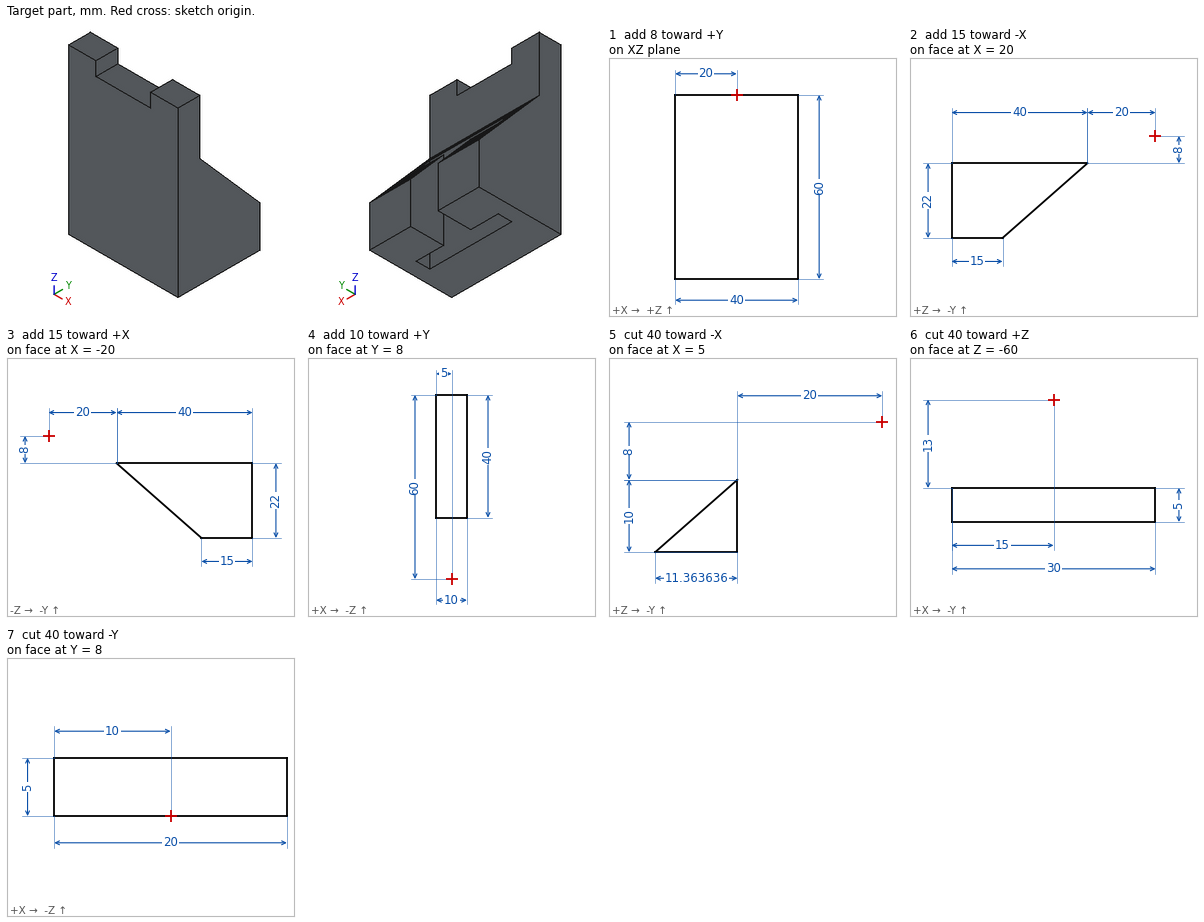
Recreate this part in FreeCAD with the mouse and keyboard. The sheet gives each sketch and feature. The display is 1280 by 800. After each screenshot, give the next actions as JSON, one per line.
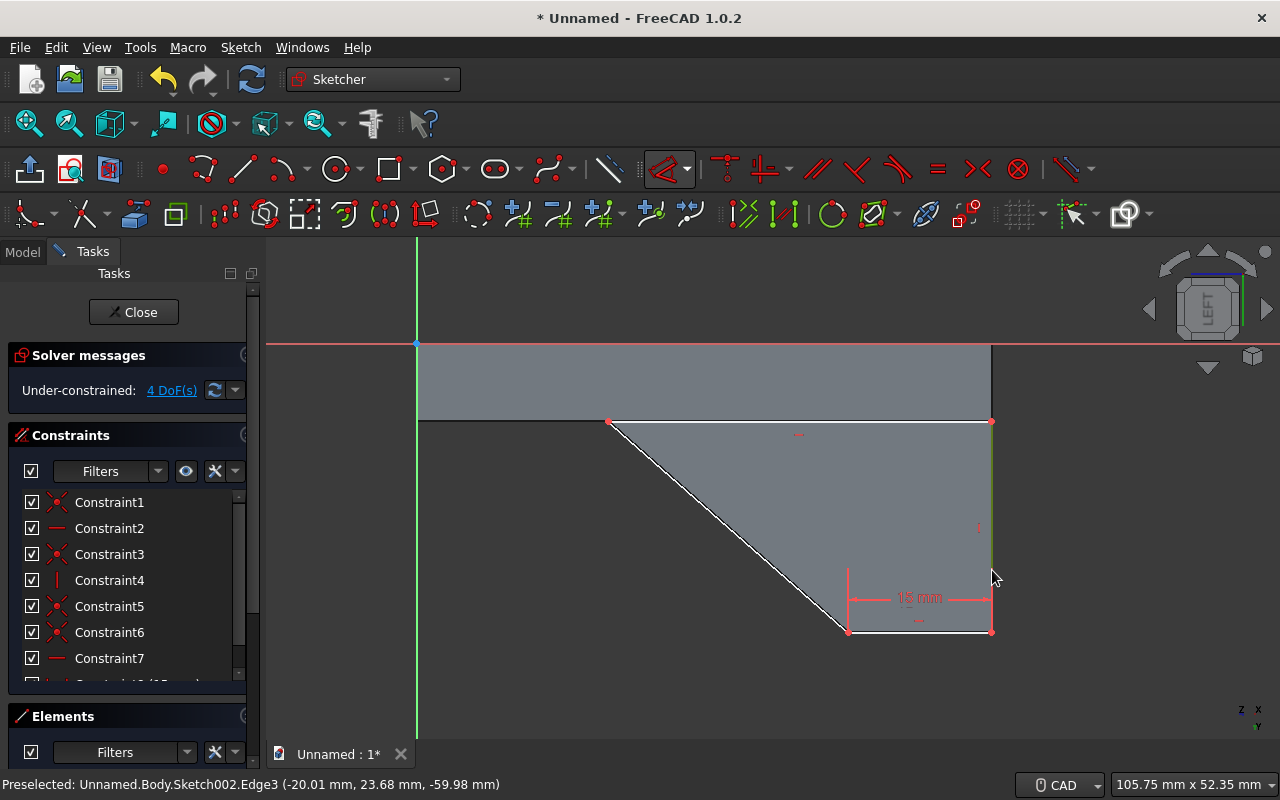
{"action": "left_click", "coordinate": [690, 170]}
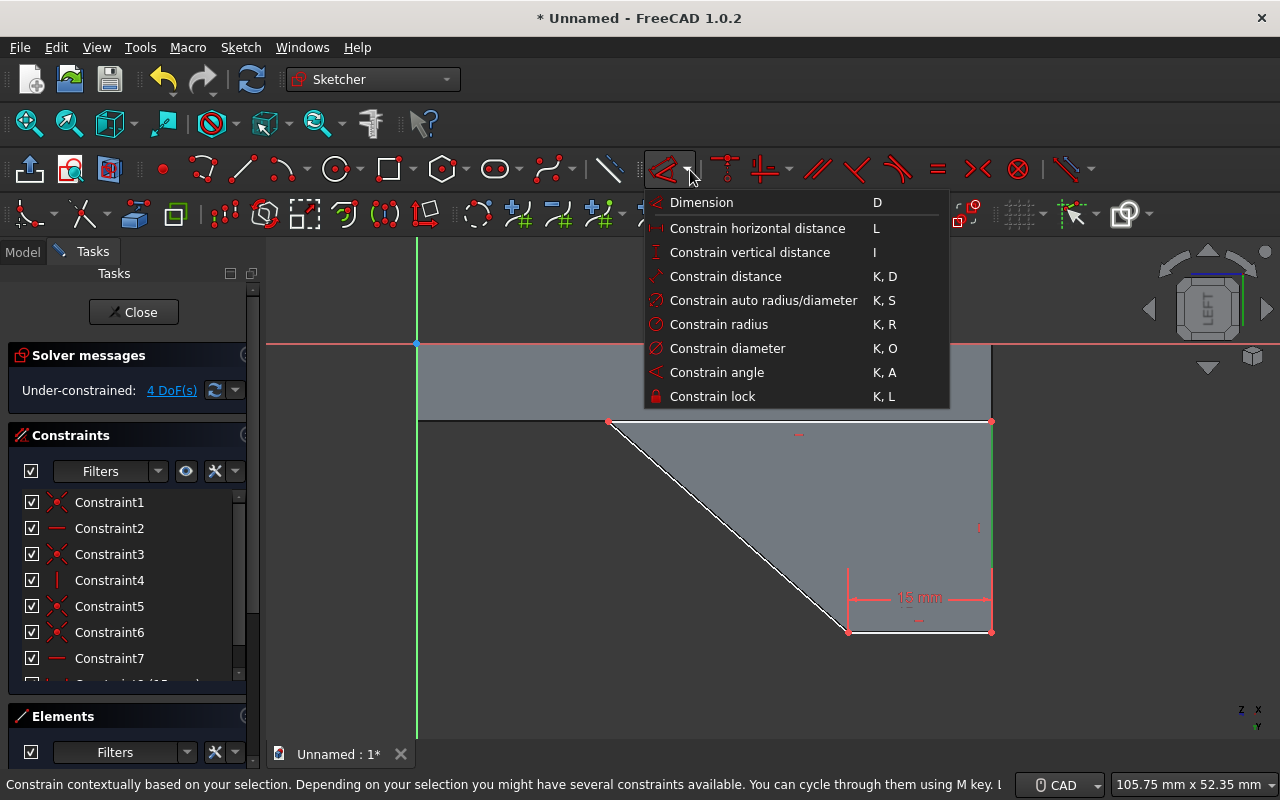
{"action": "left_click", "coordinate": [797, 252]}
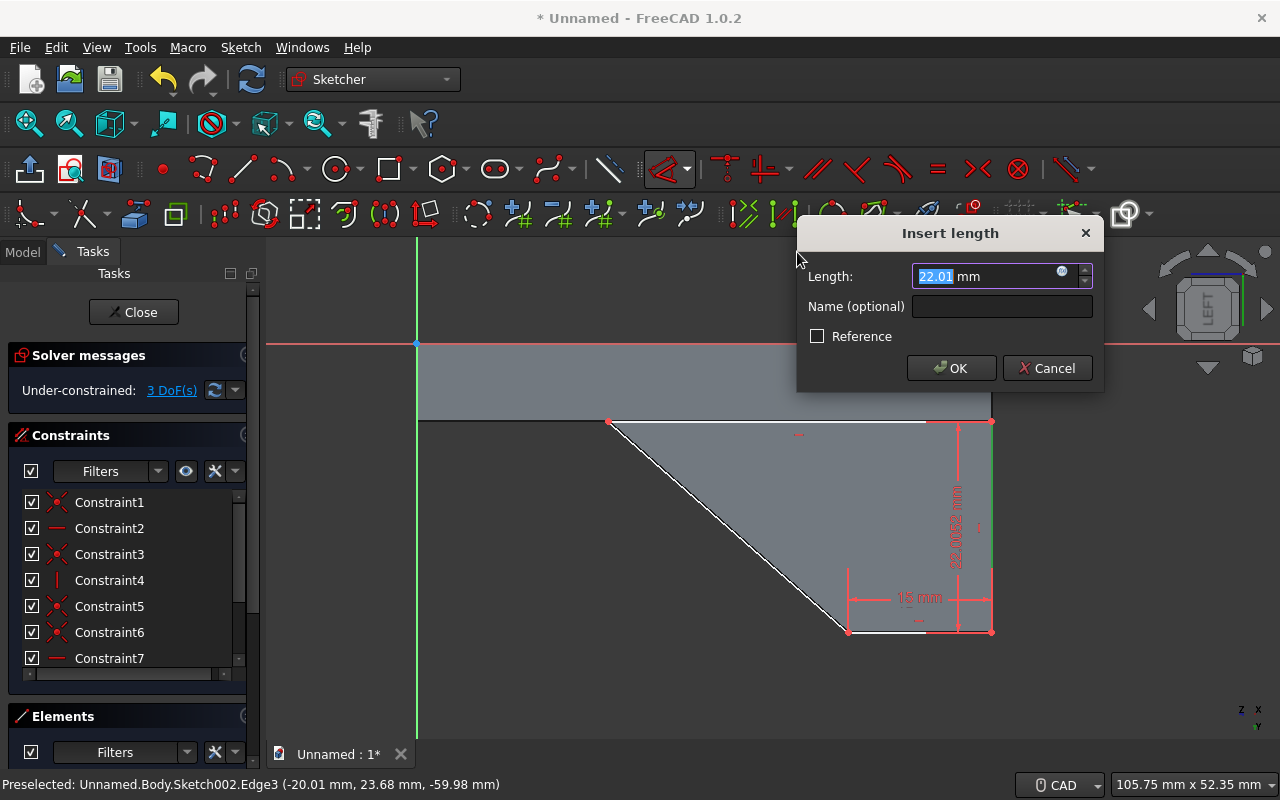
{"action": "type", "text": "22"}
{"action": "key", "text": "Return"}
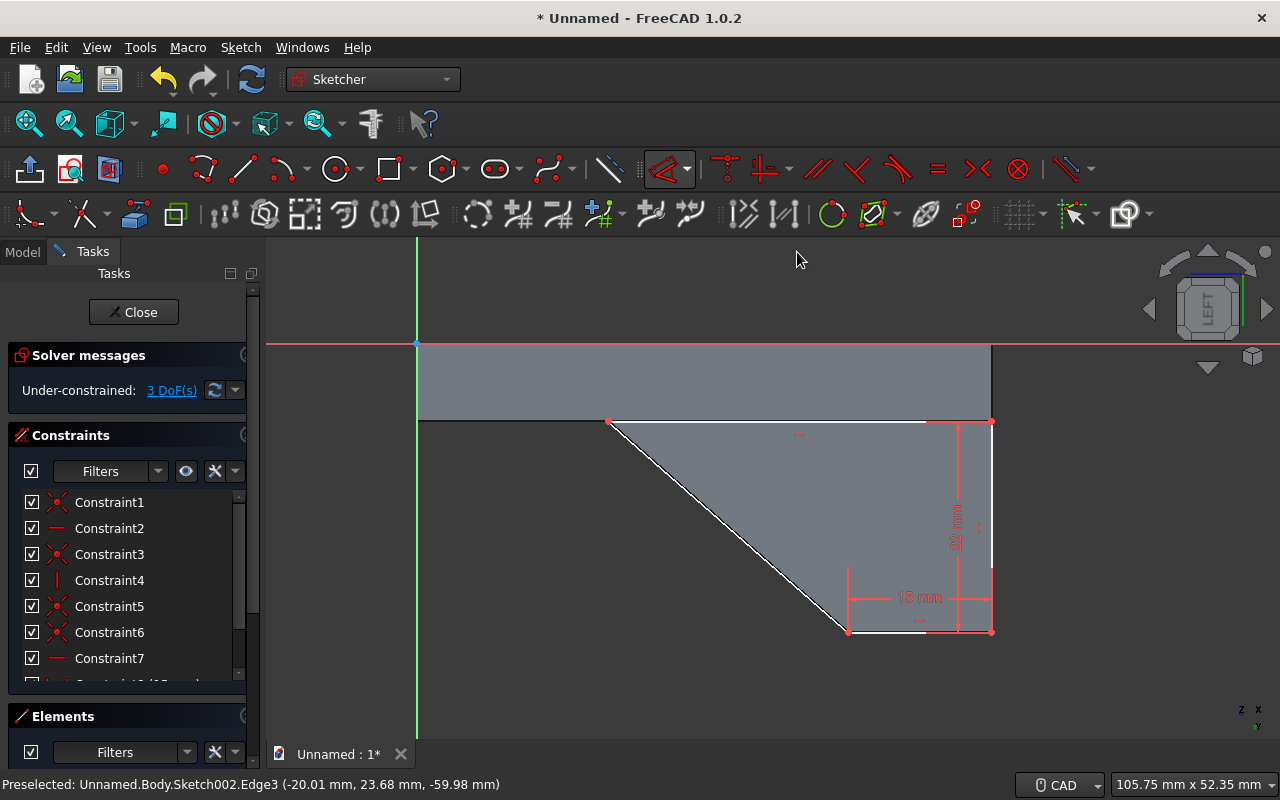
{"action": "left_click", "coordinate": [877, 422]}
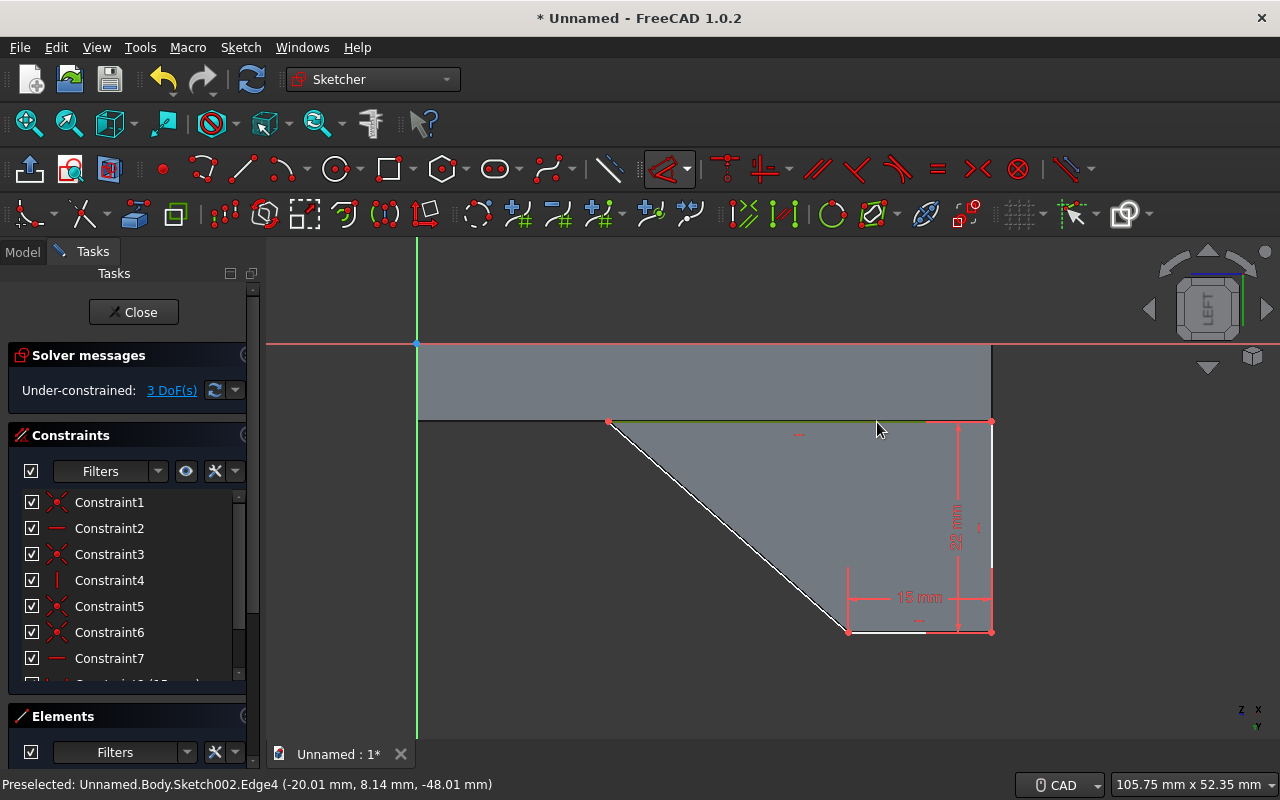
{"action": "left_click", "coordinate": [690, 170]}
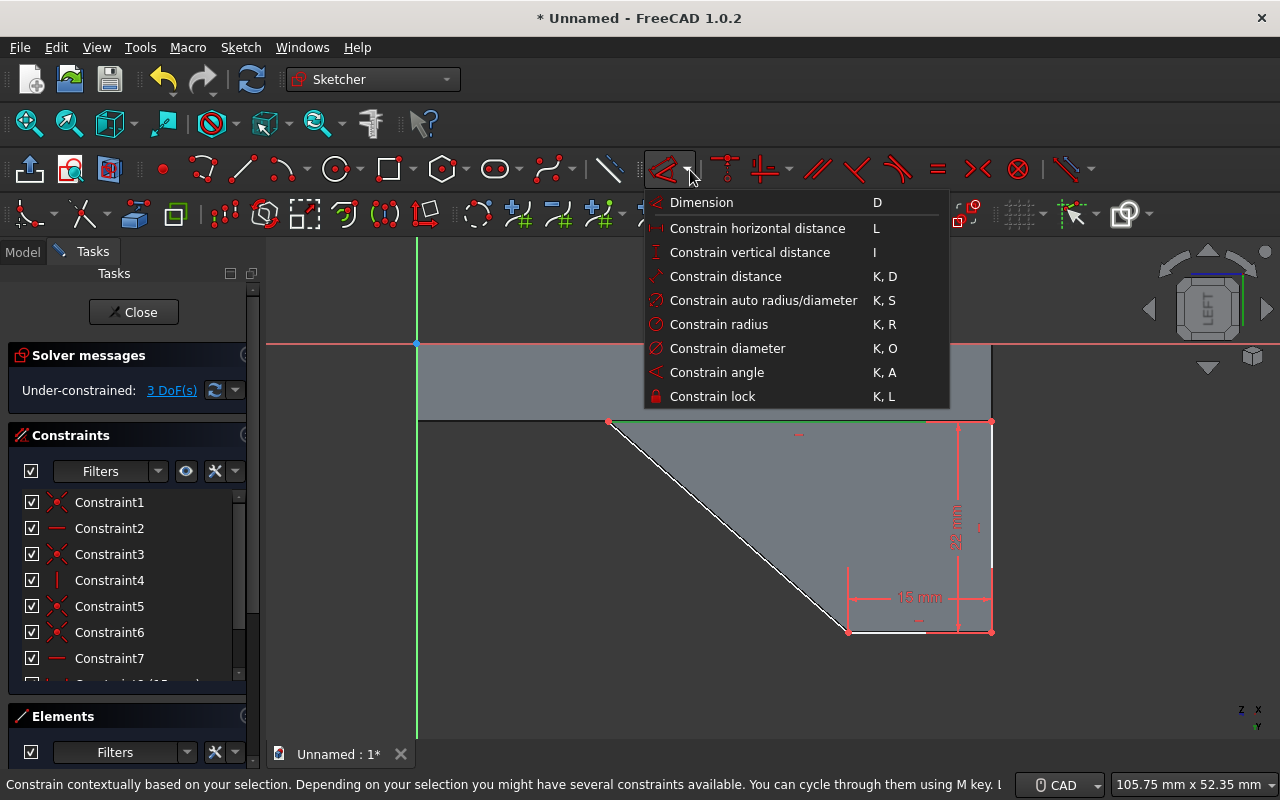
{"action": "left_click", "coordinate": [797, 228]}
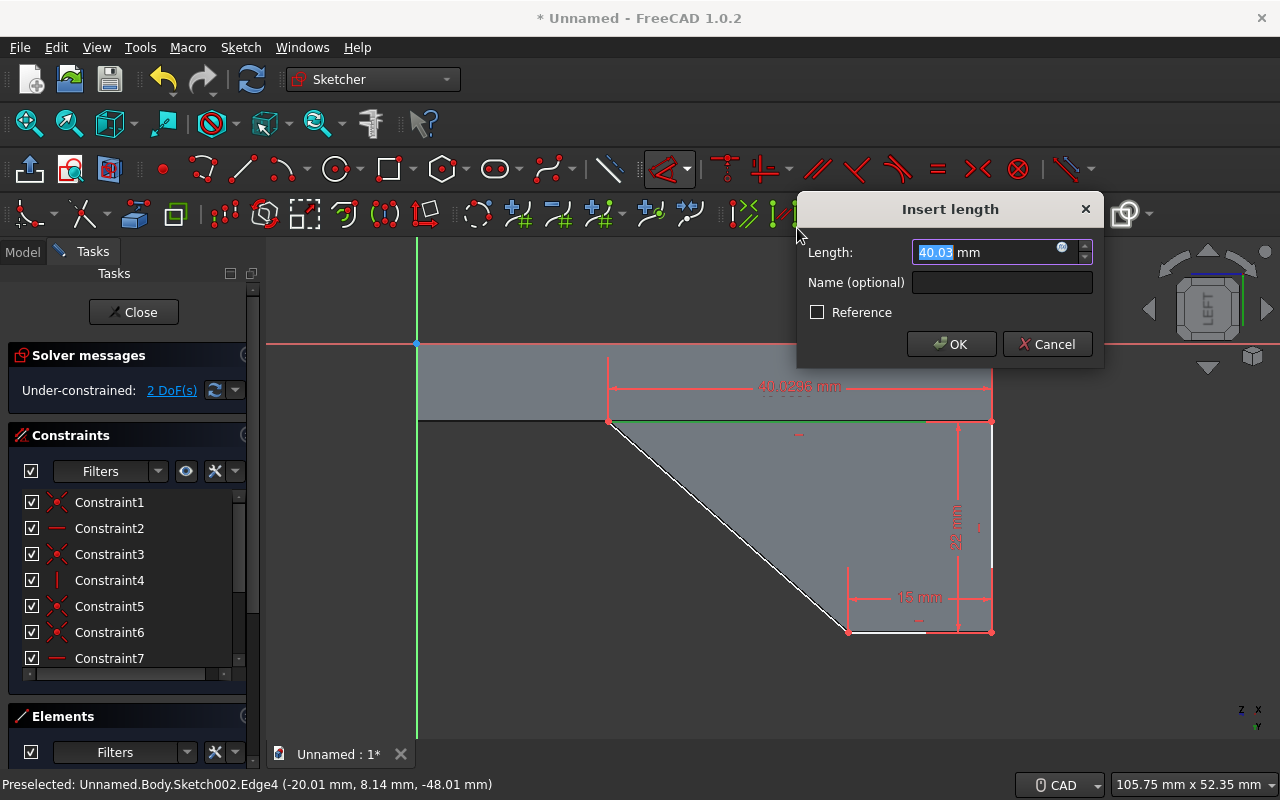
{"action": "type", "text": "40"}
{"action": "key", "text": "Return"}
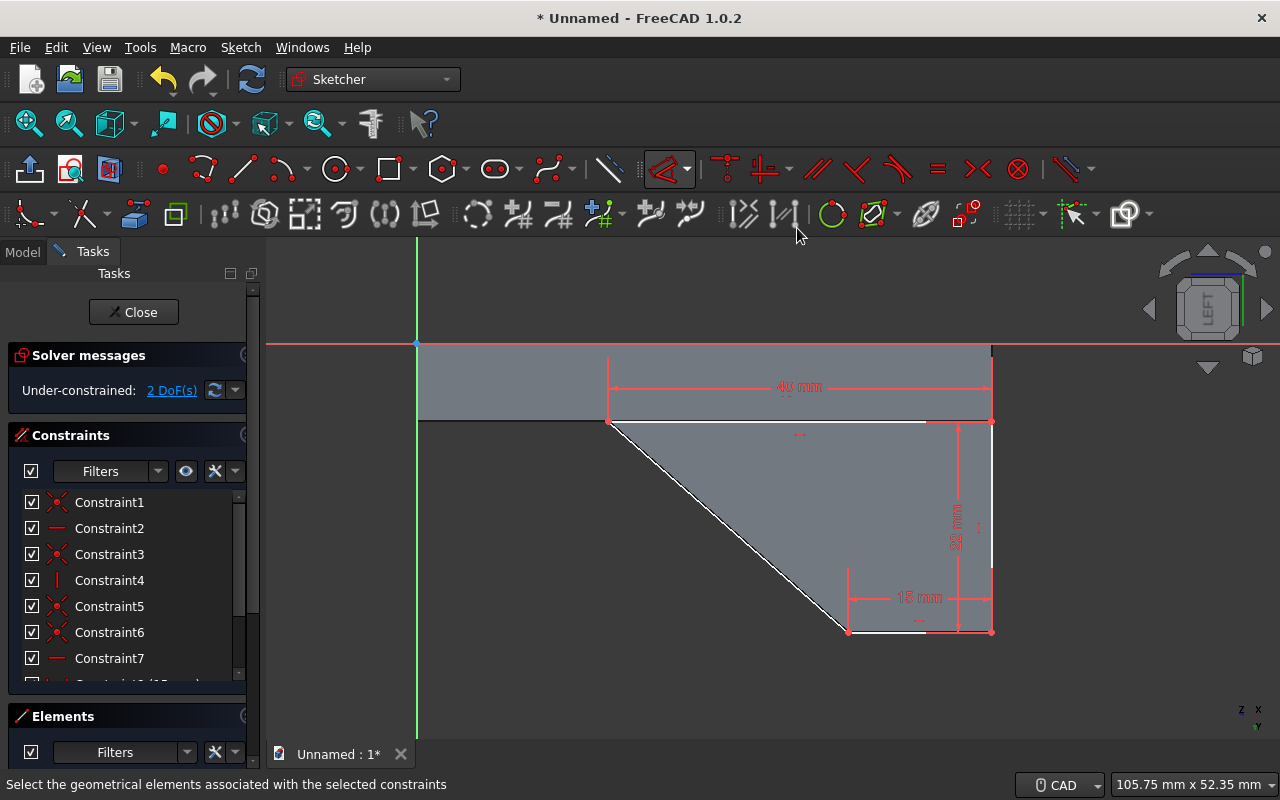
{"action": "left_click", "coordinate": [608, 422]}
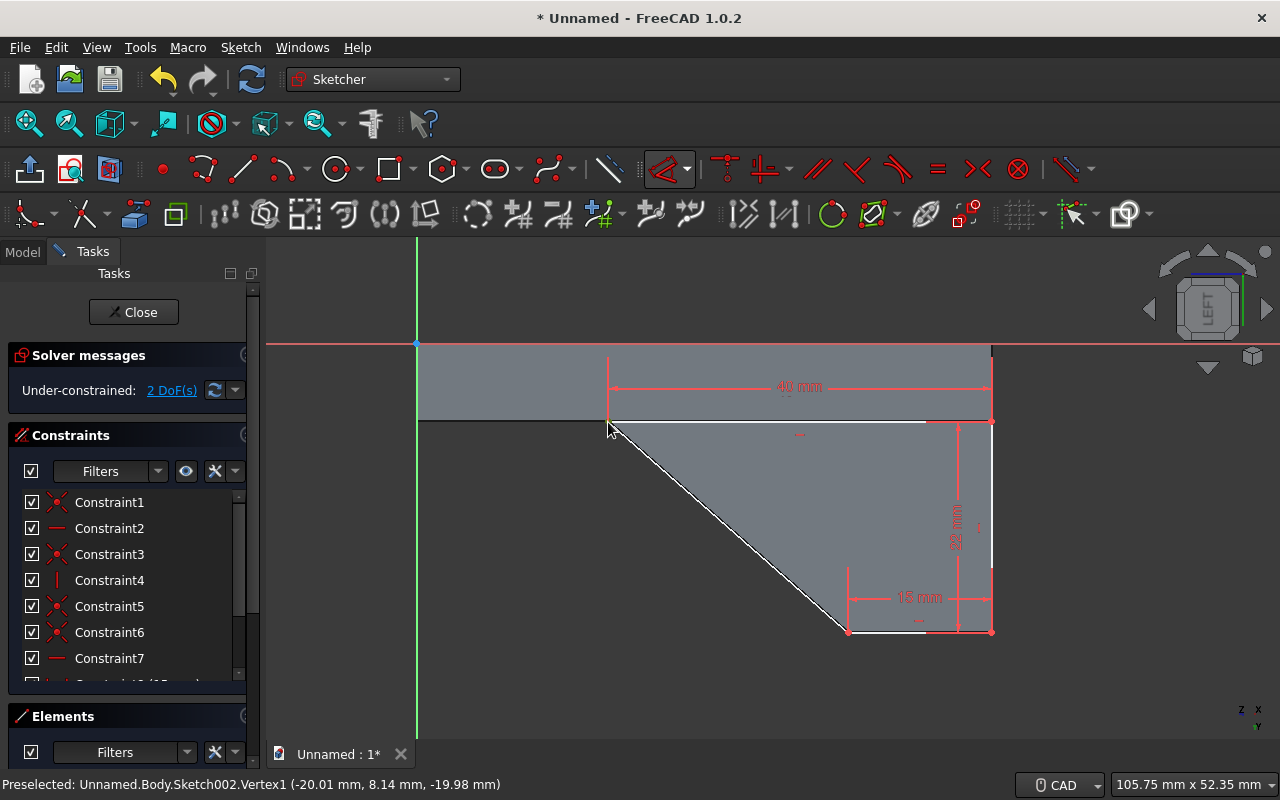
{"action": "left_click", "coordinate": [690, 170]}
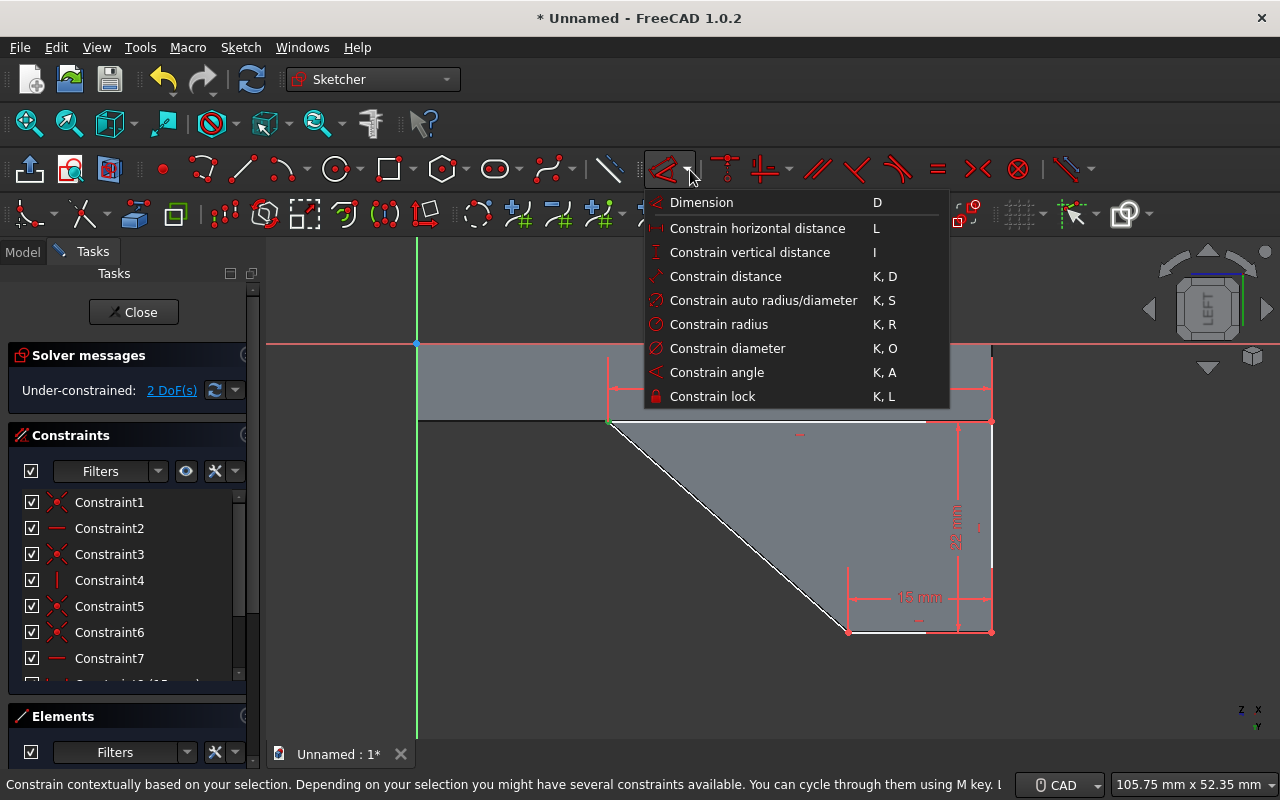
{"action": "left_click", "coordinate": [797, 252]}